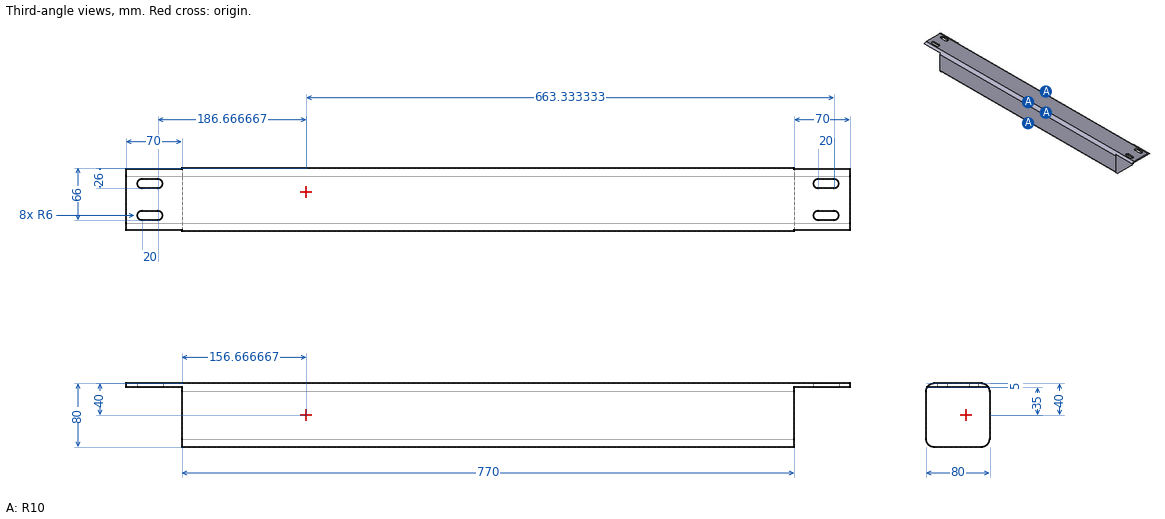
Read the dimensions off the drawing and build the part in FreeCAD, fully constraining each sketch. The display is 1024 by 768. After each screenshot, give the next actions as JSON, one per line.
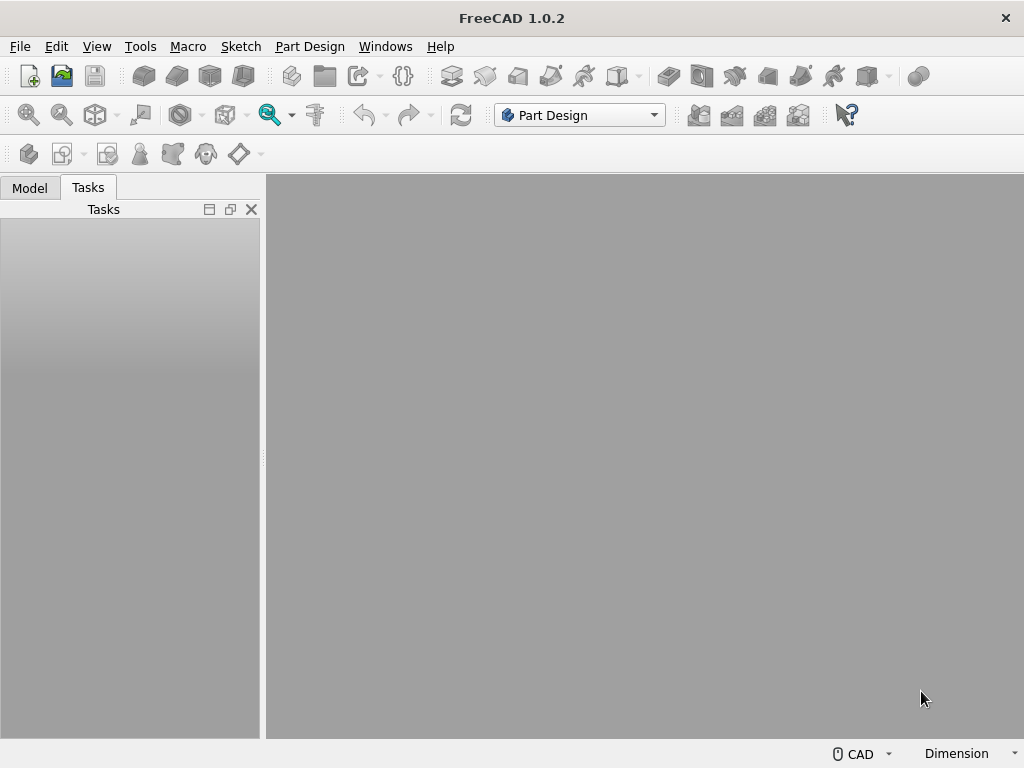
{"action": "left_click", "coordinate": [29, 76]}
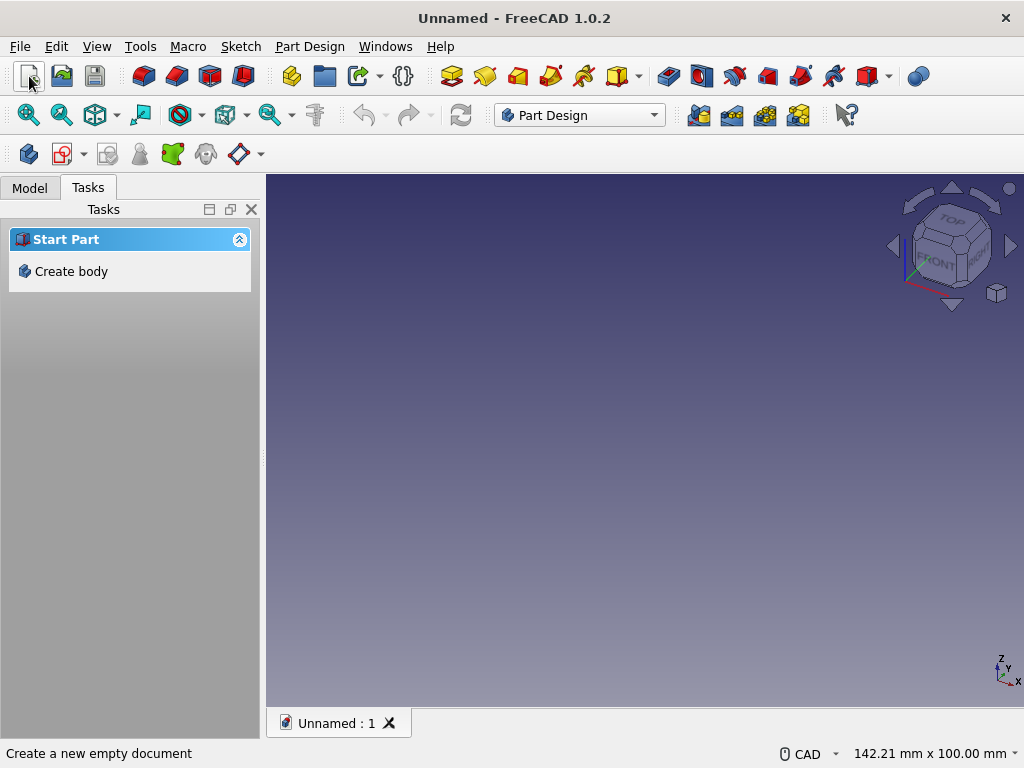
{"action": "left_click", "coordinate": [29, 154]}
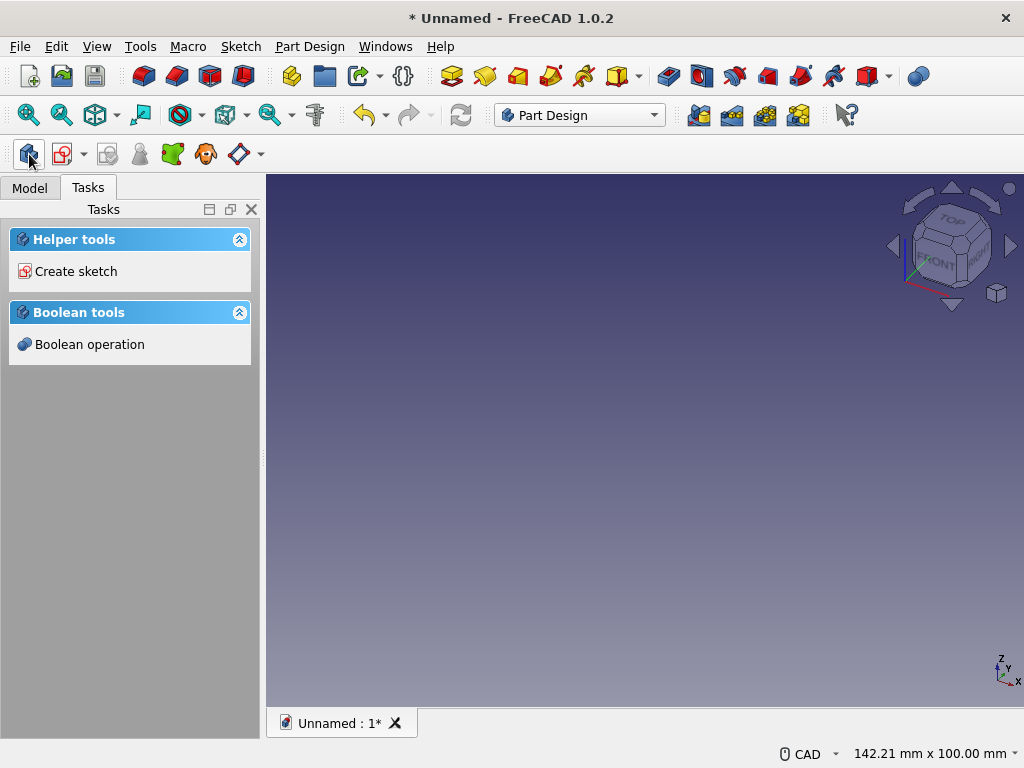
{"action": "left_click", "coordinate": [30, 188]}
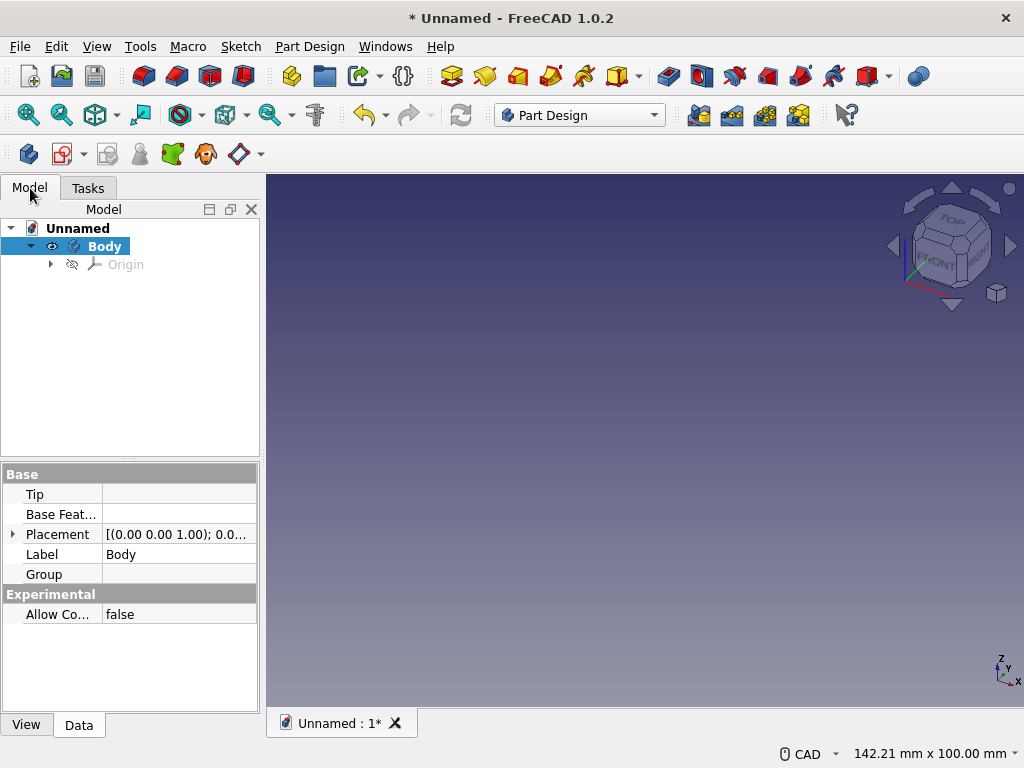
{"action": "left_click", "coordinate": [51, 264]}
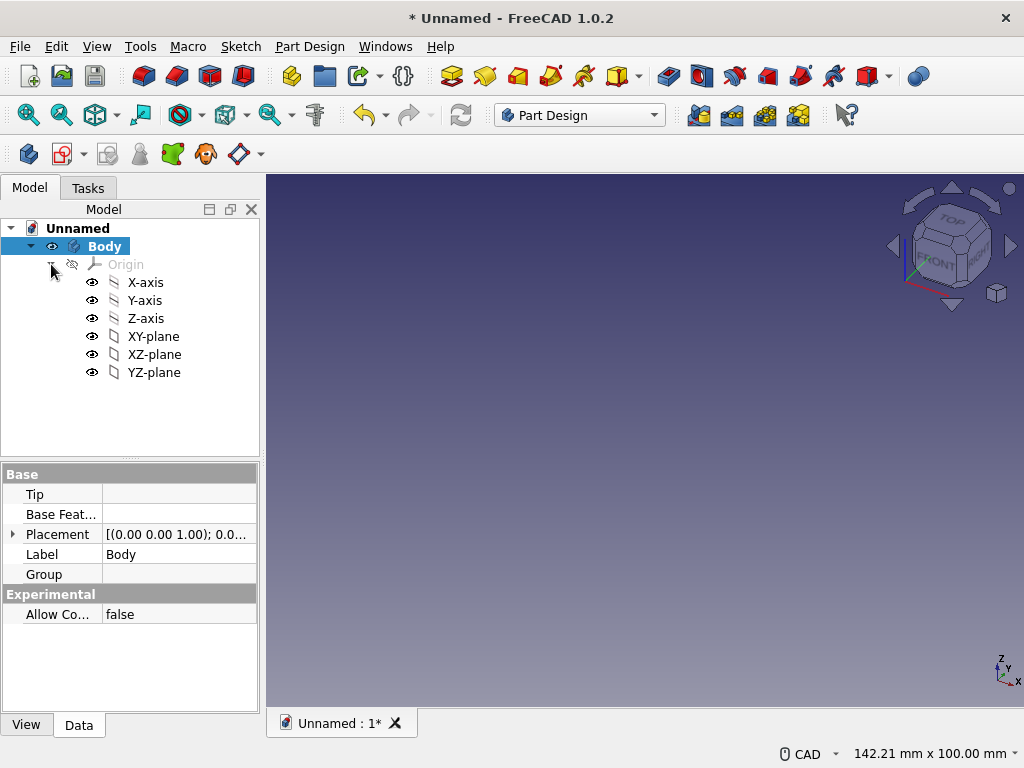
{"action": "left_click", "coordinate": [137, 354]}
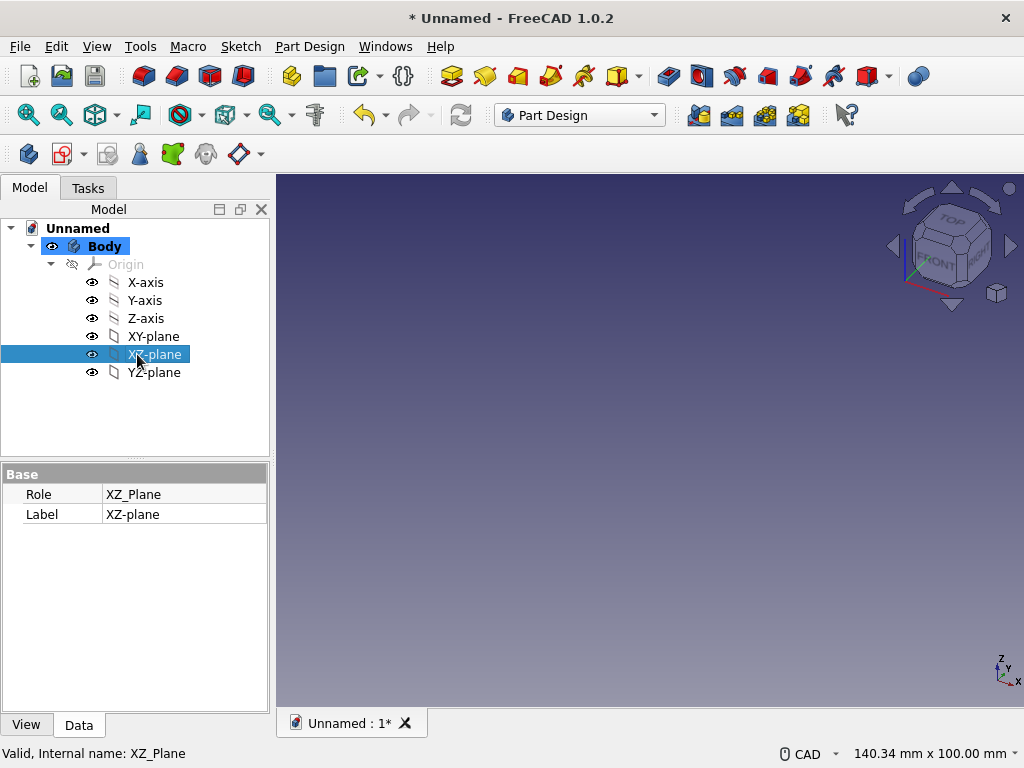
{"action": "left_click", "coordinate": [238, 154]}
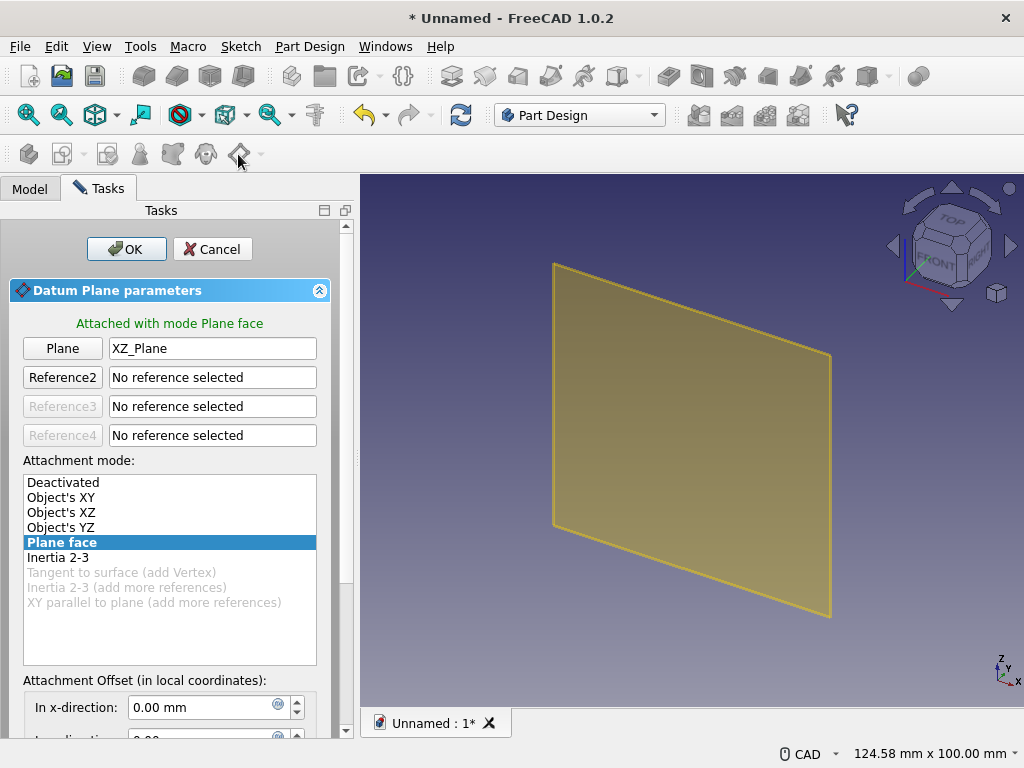
{"action": "scroll", "coordinate": [346, 479], "scroll_direction": "down", "scroll_amount": 2}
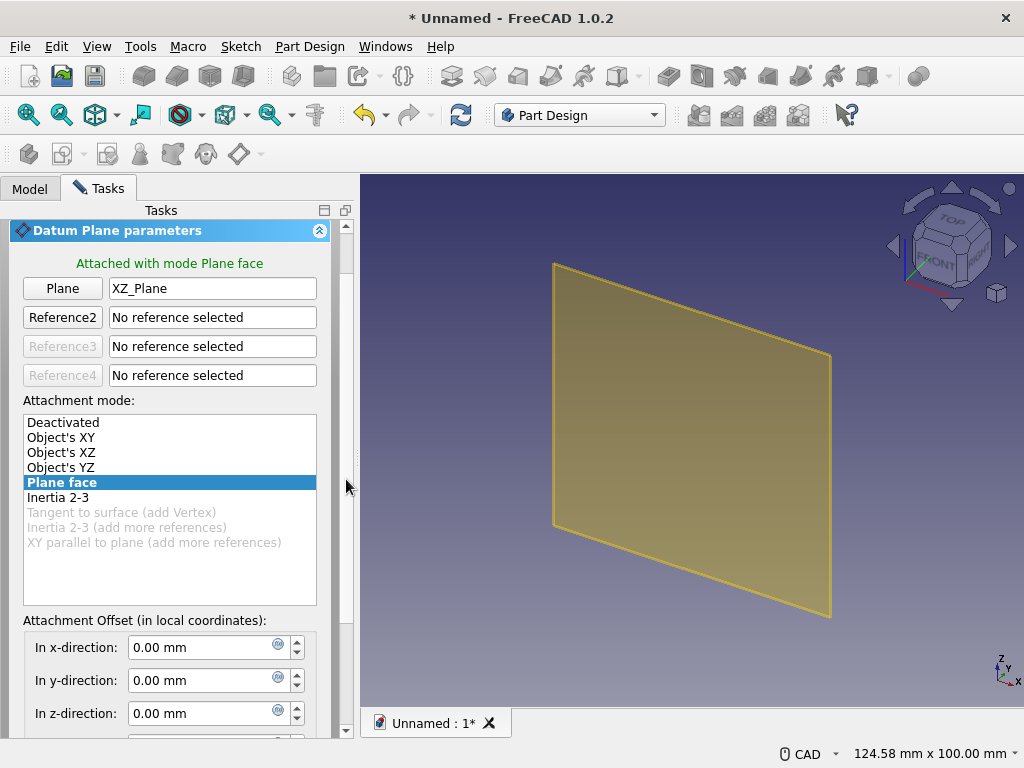
{"action": "triple_click", "coordinate": [210, 654]}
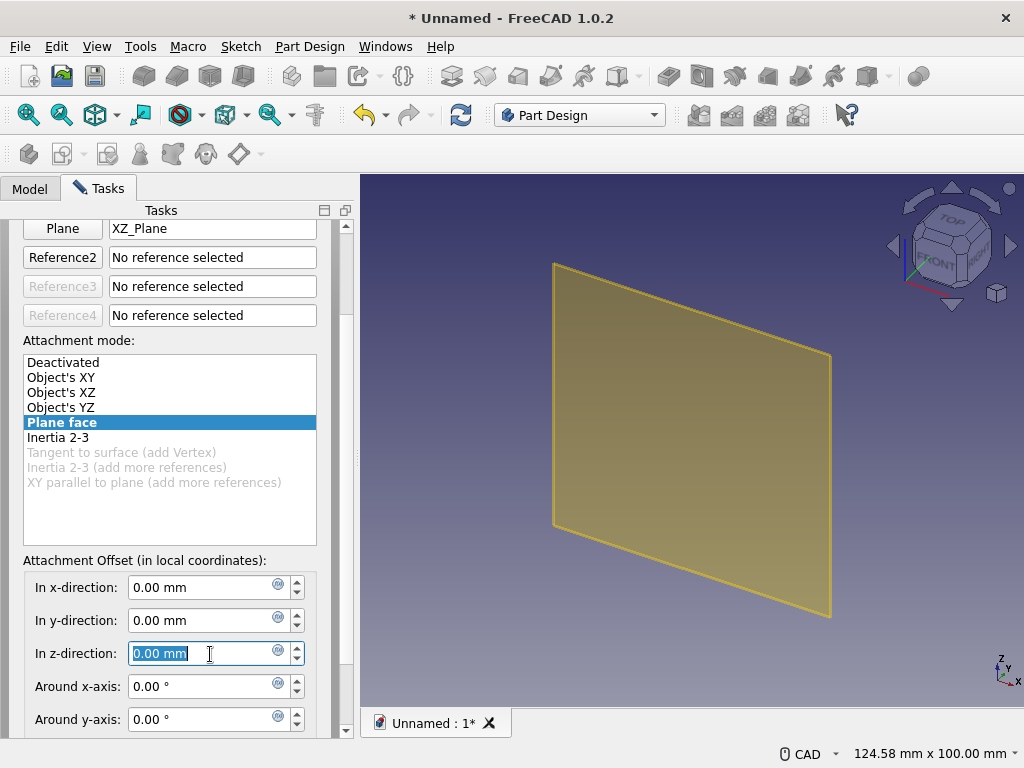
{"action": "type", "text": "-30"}
{"action": "key", "text": "Tab"}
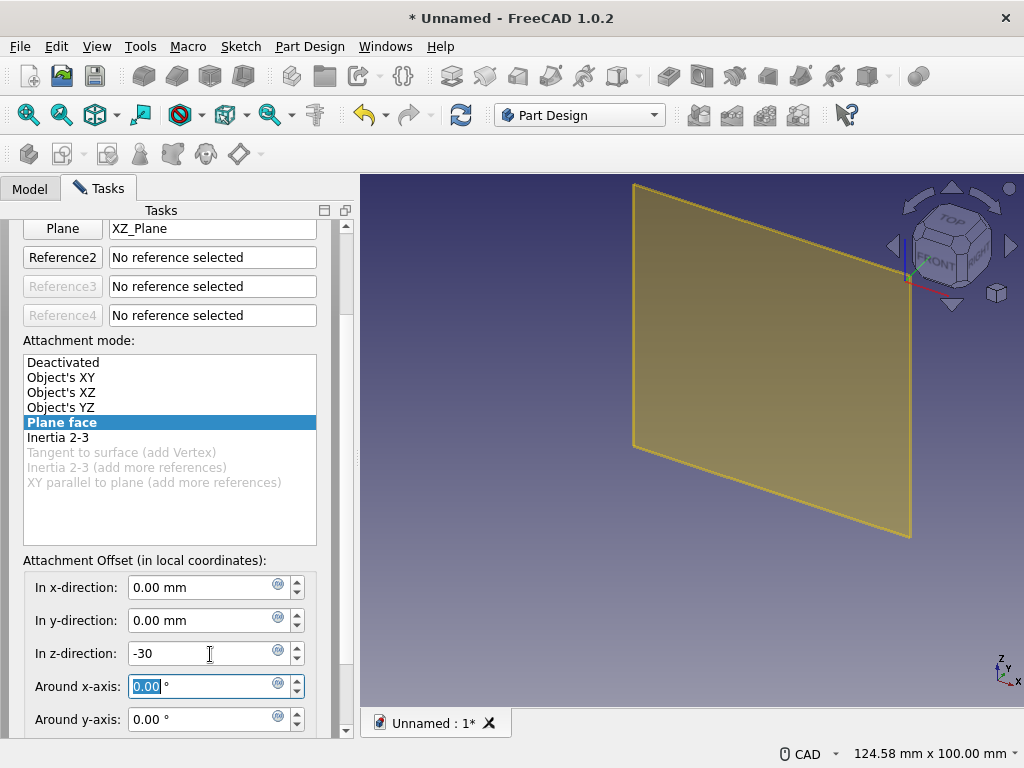
{"action": "scroll", "coordinate": [346, 479], "scroll_direction": "up", "scroll_amount": 3}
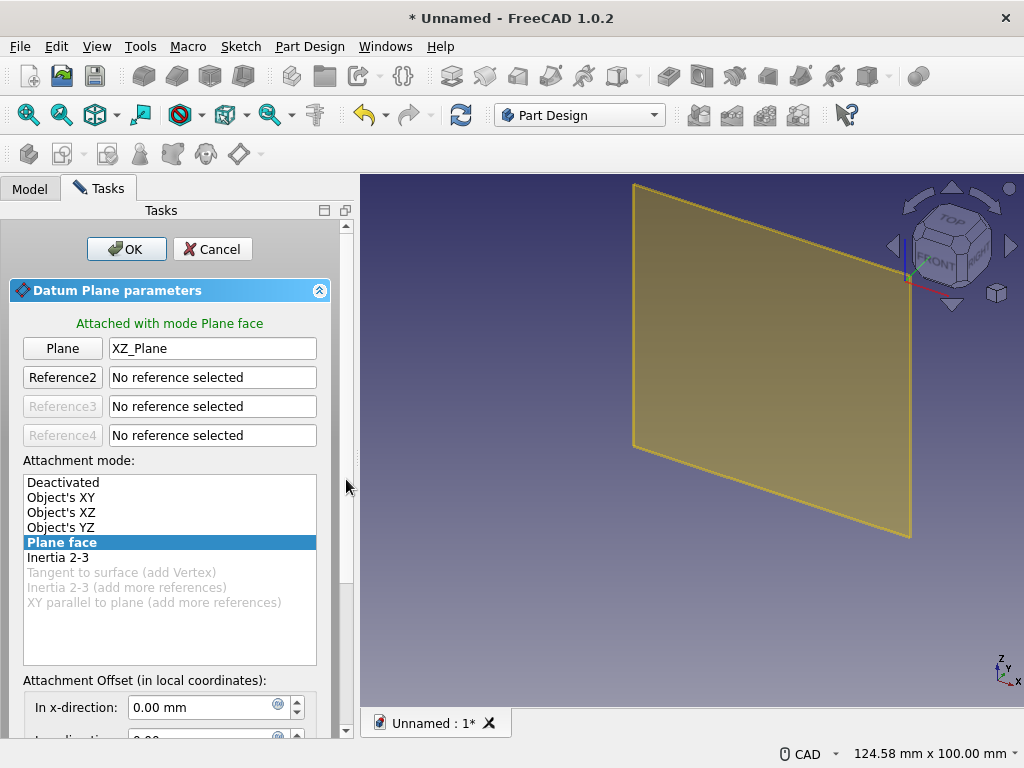
{"action": "left_click", "coordinate": [127, 249]}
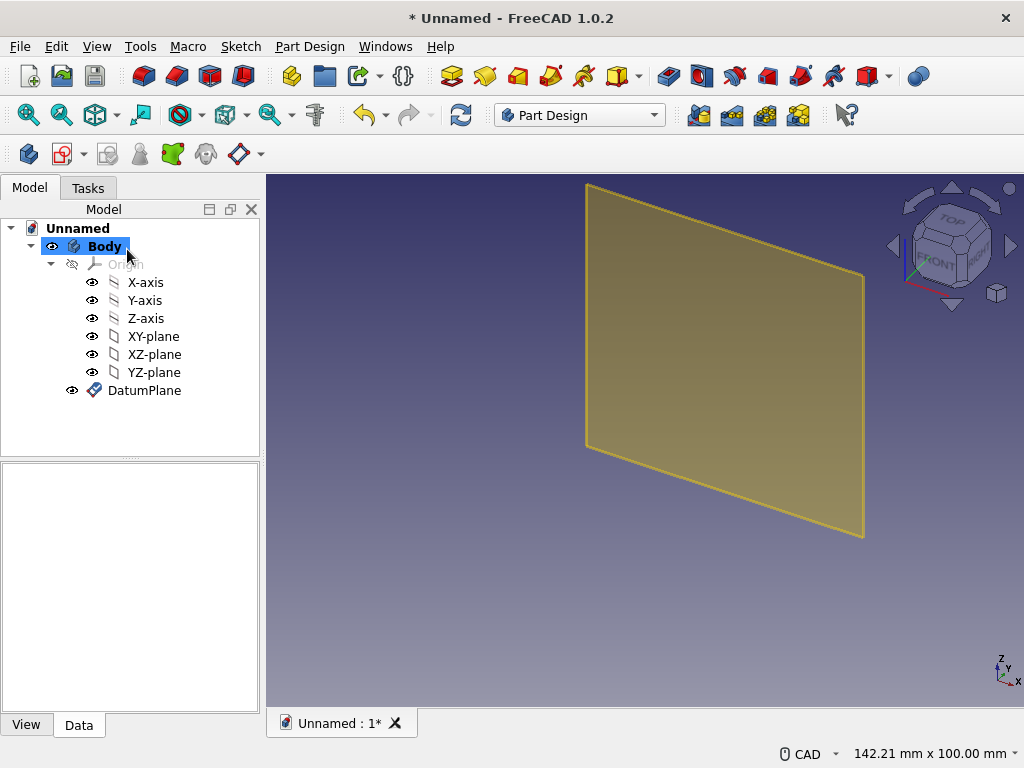
{"action": "left_click", "coordinate": [117, 390]}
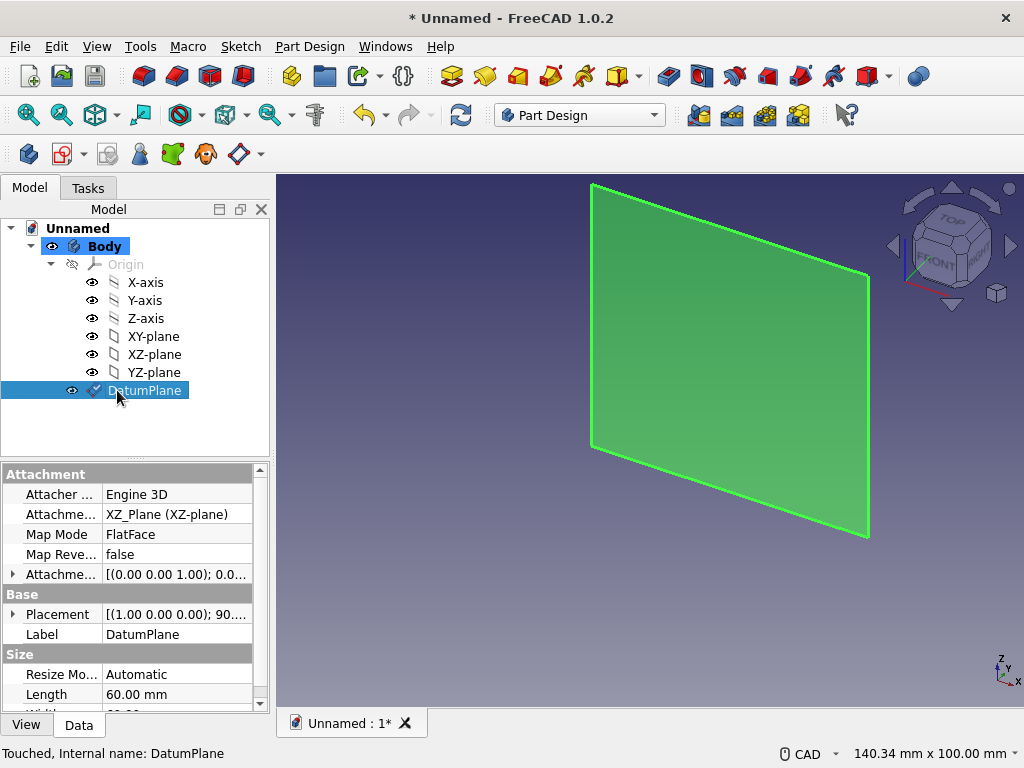
{"action": "left_click", "coordinate": [62, 154]}